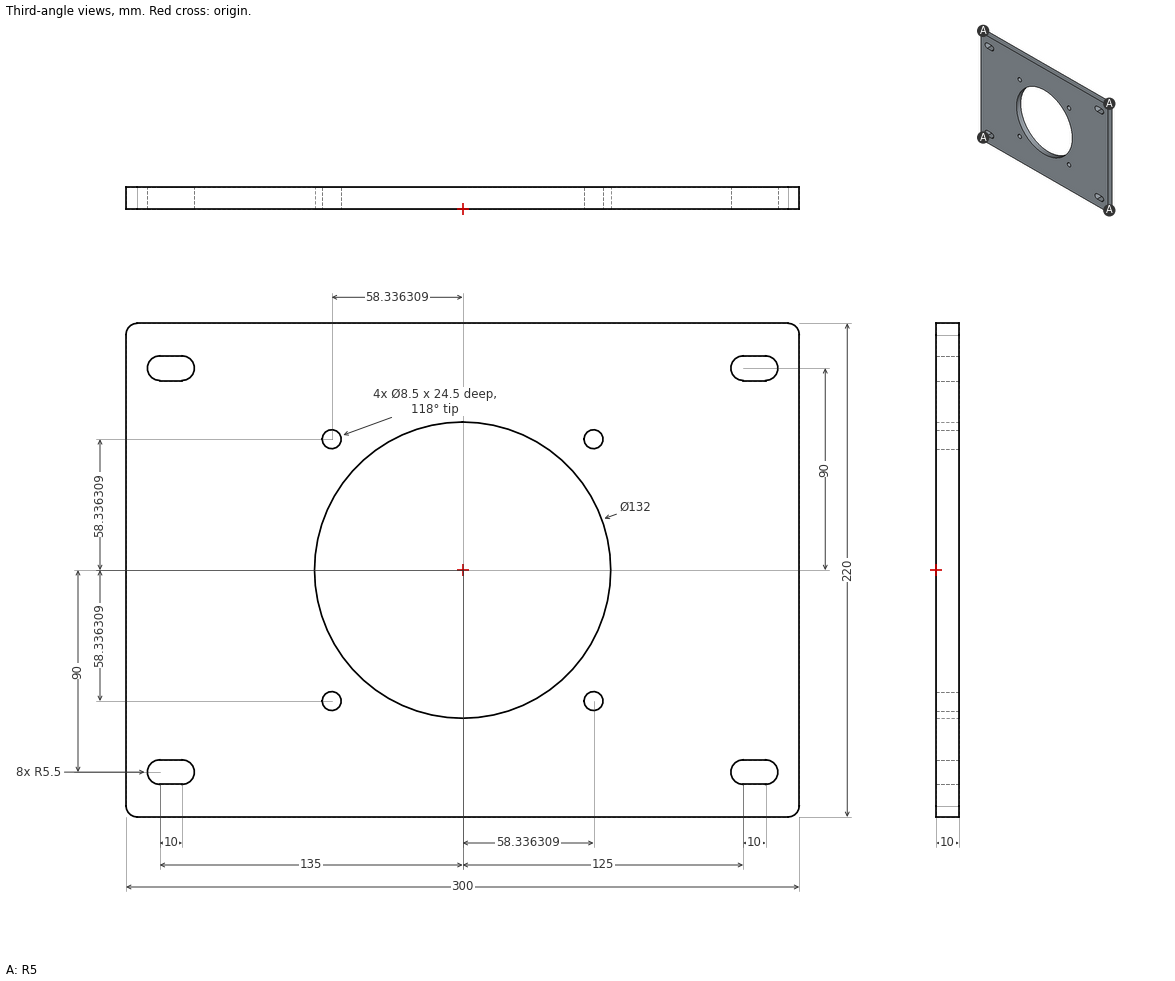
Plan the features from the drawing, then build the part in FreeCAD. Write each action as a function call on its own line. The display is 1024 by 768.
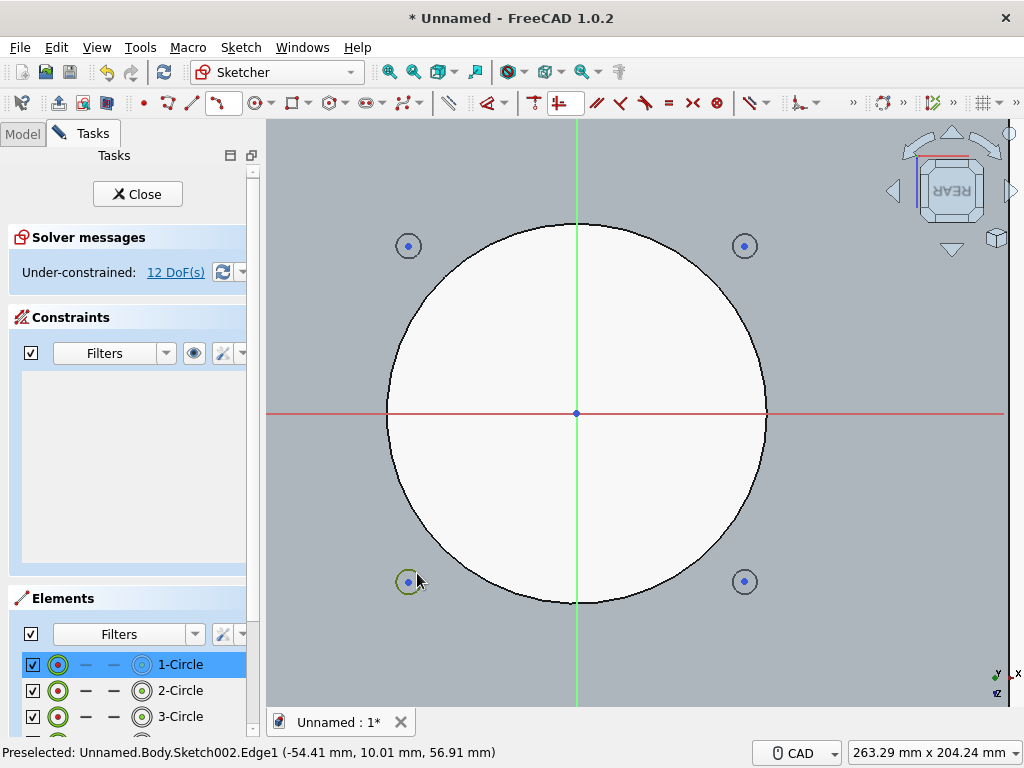
click(417, 237)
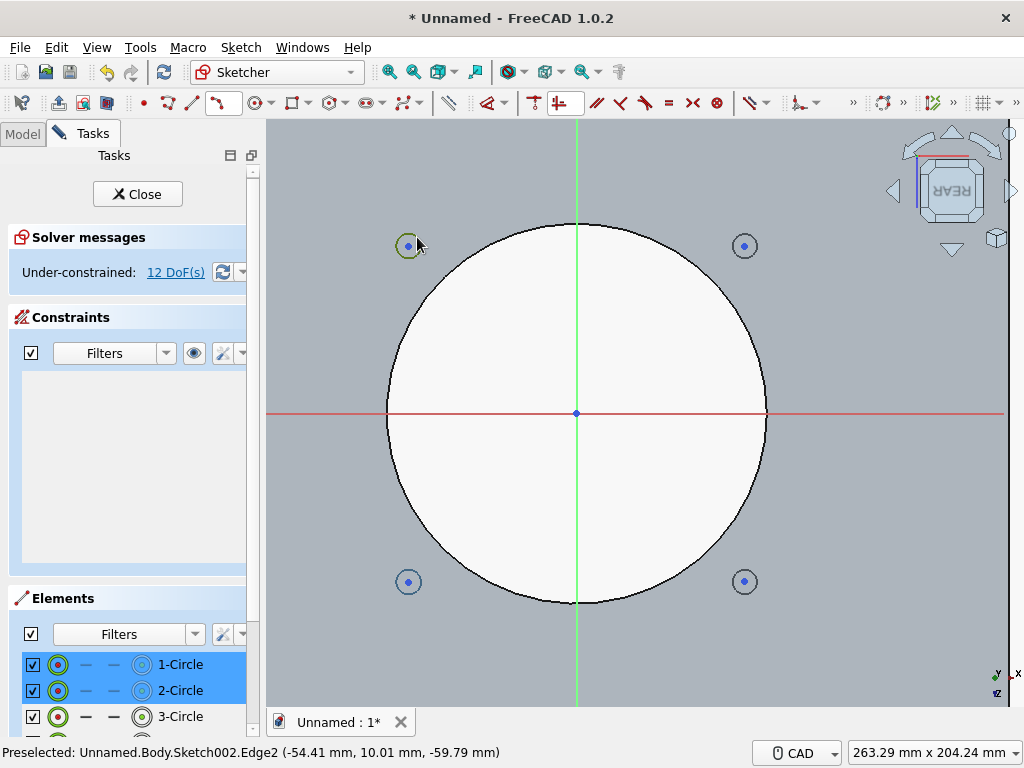
click(753, 238)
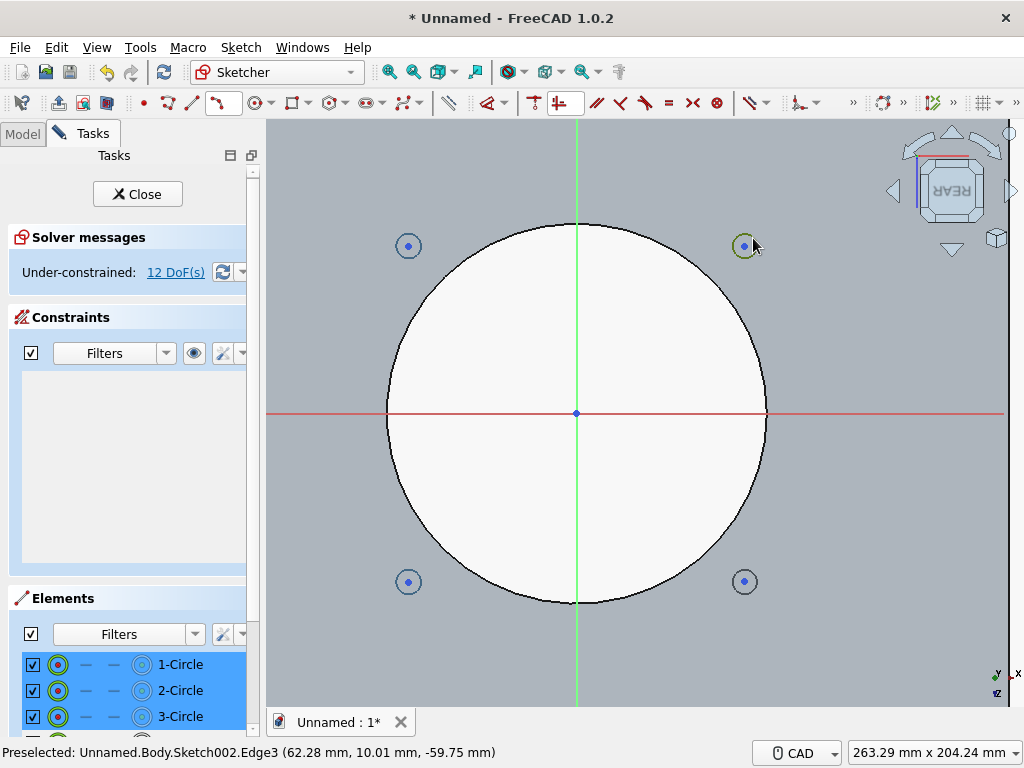
click(753, 573)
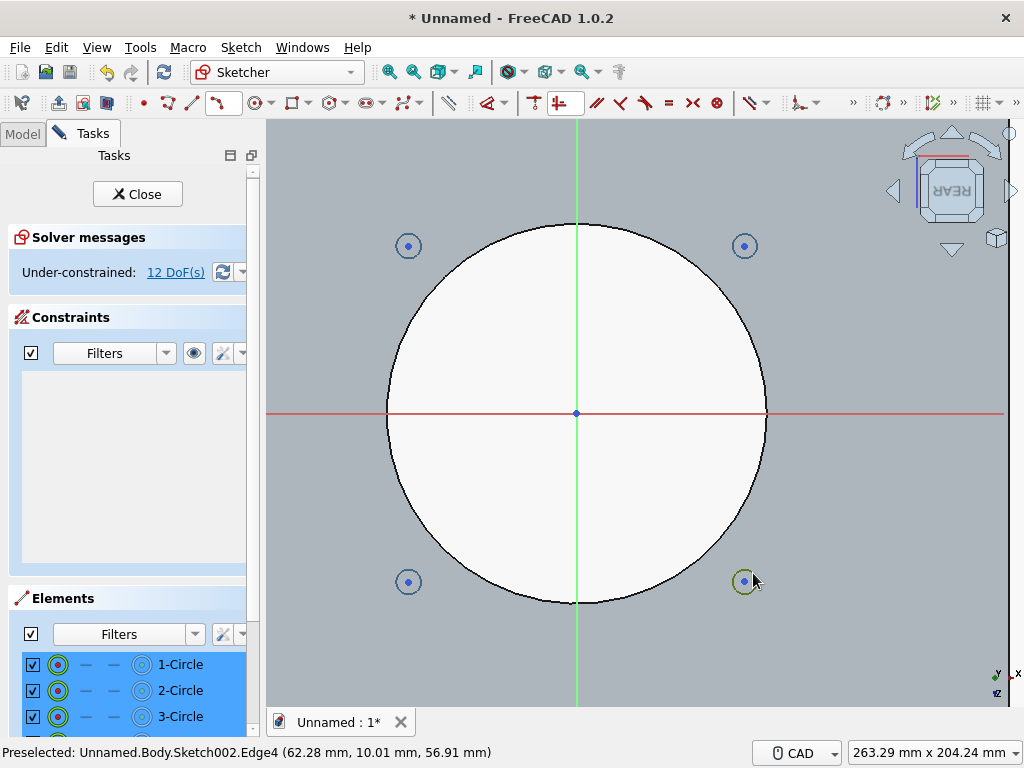
key(e)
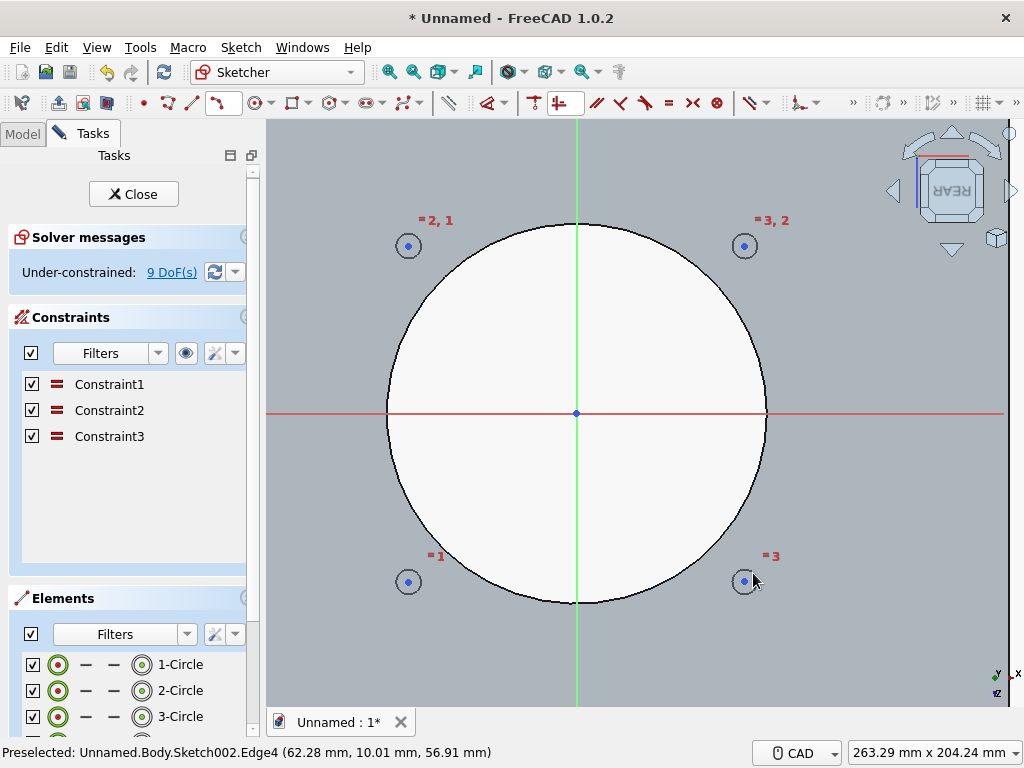
click(409, 582)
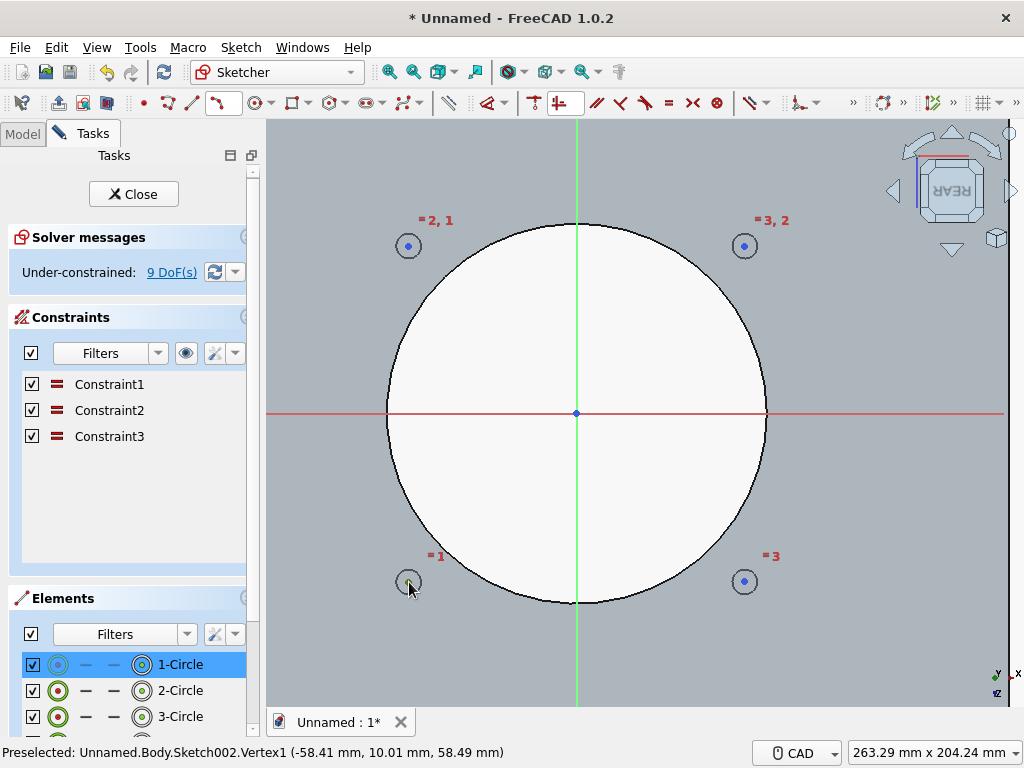
click(409, 246)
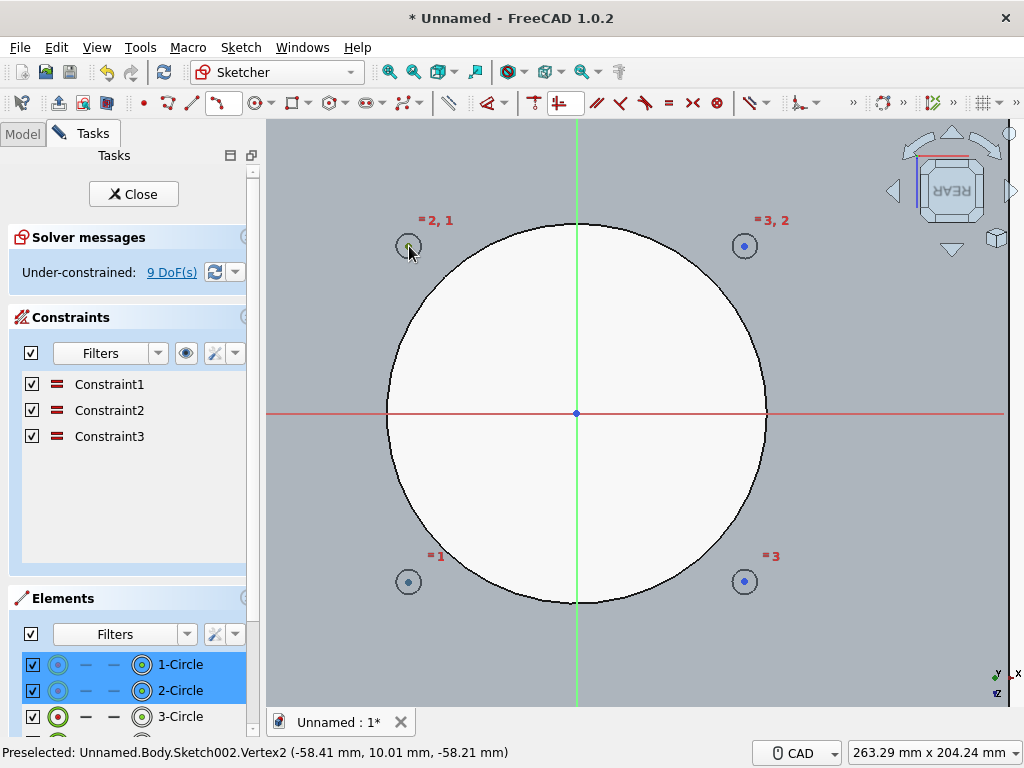
key(v)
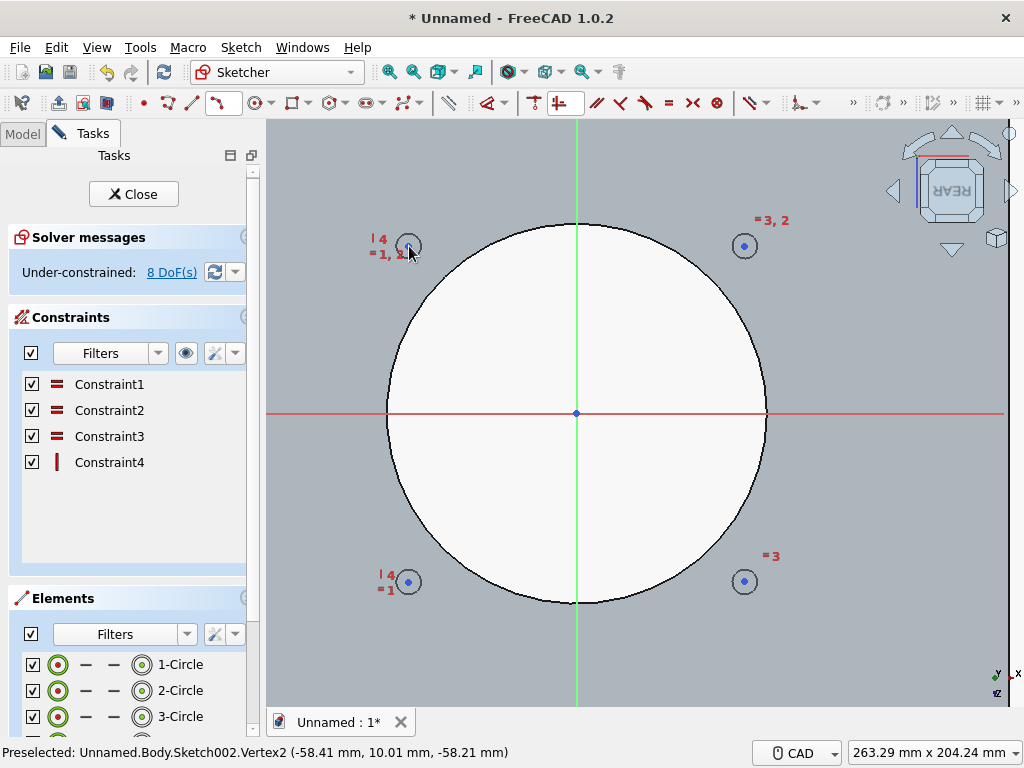
click(409, 246)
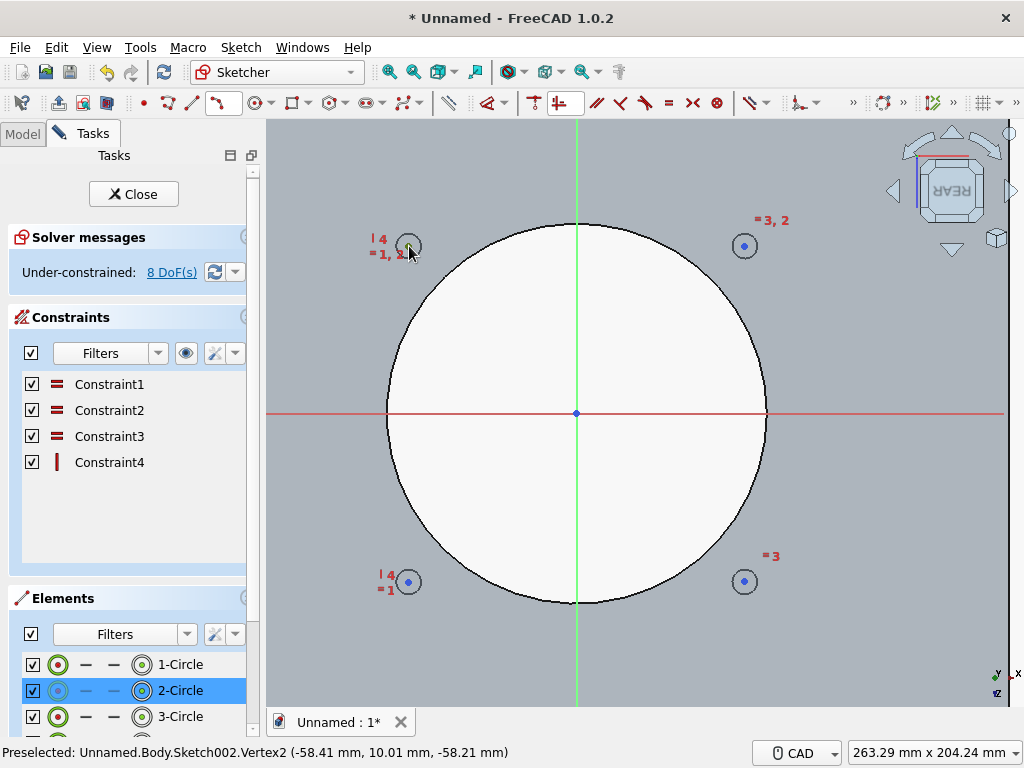
click(745, 246)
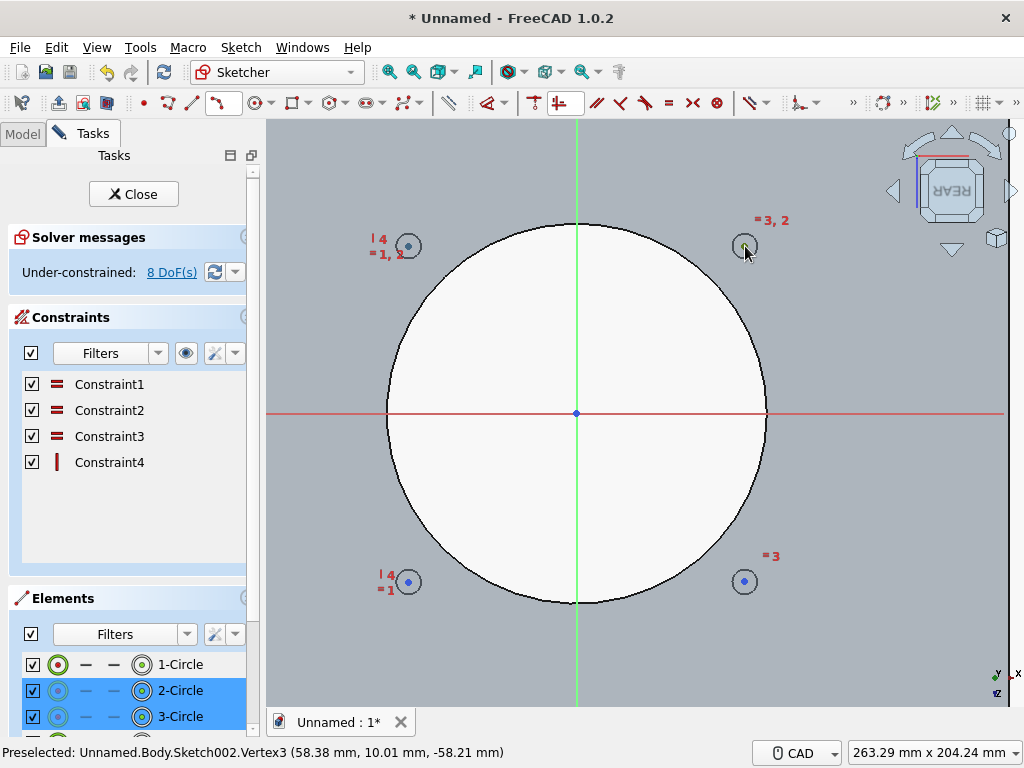
key(h)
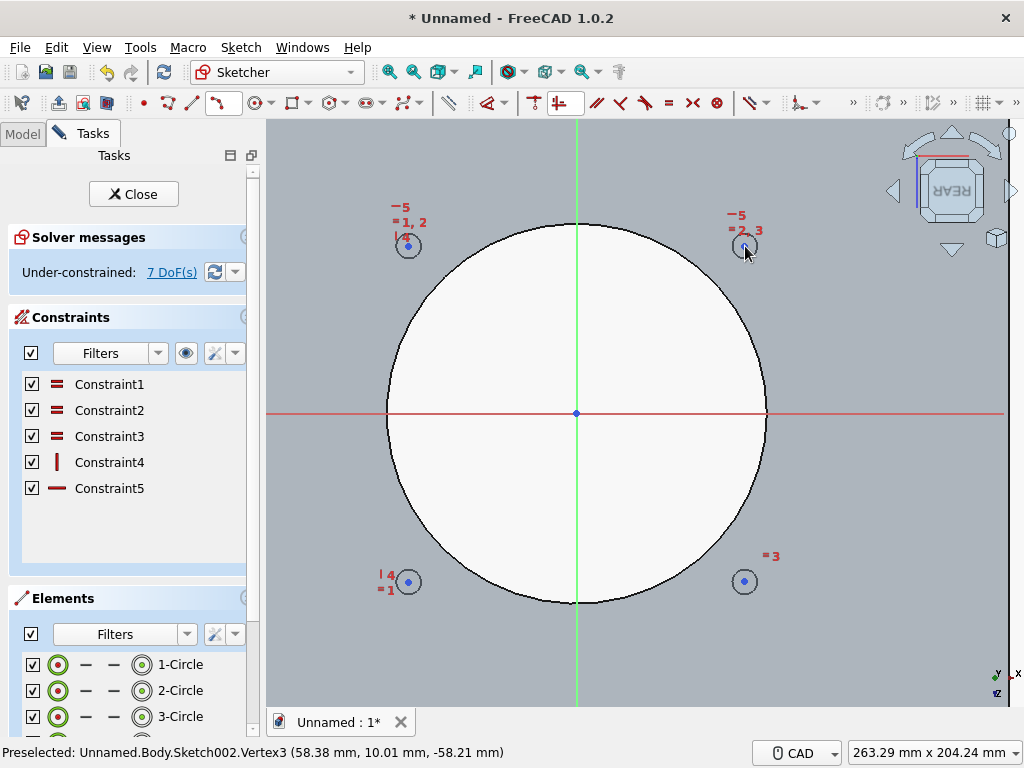
click(745, 246)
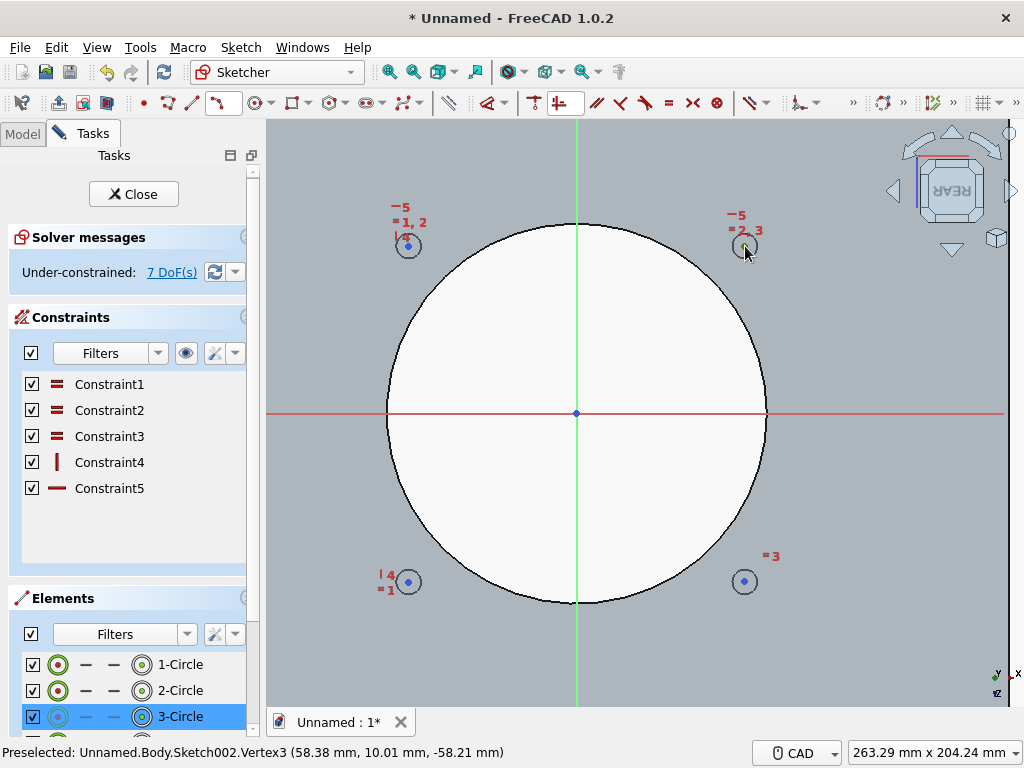
click(745, 582)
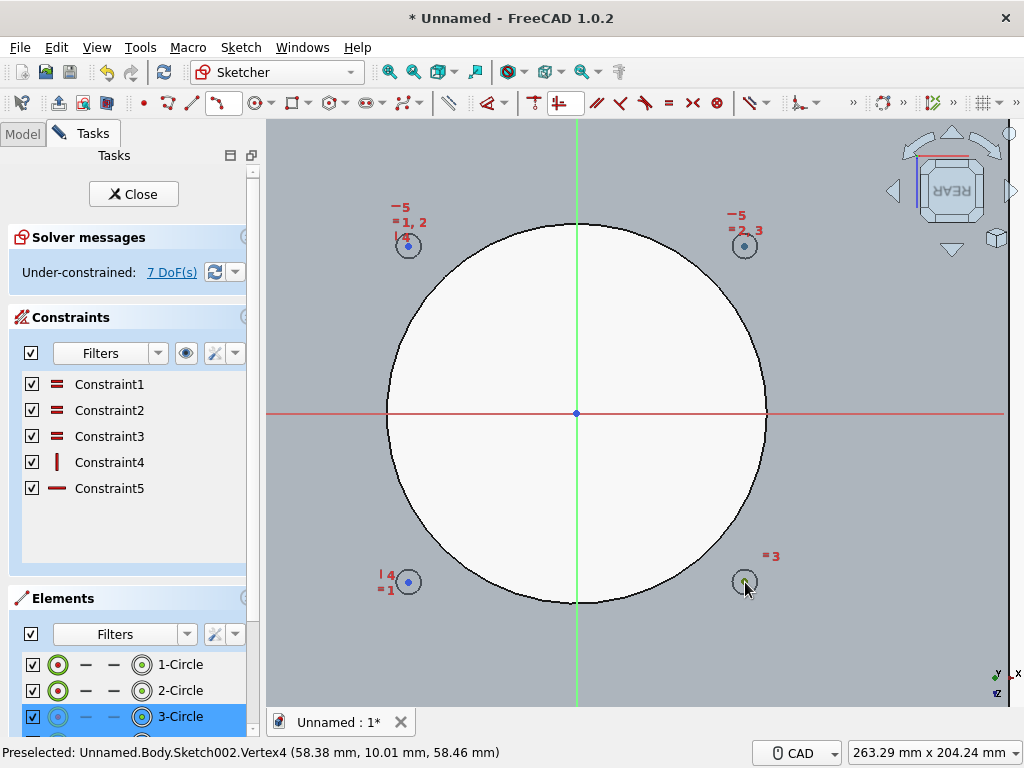
key(v)